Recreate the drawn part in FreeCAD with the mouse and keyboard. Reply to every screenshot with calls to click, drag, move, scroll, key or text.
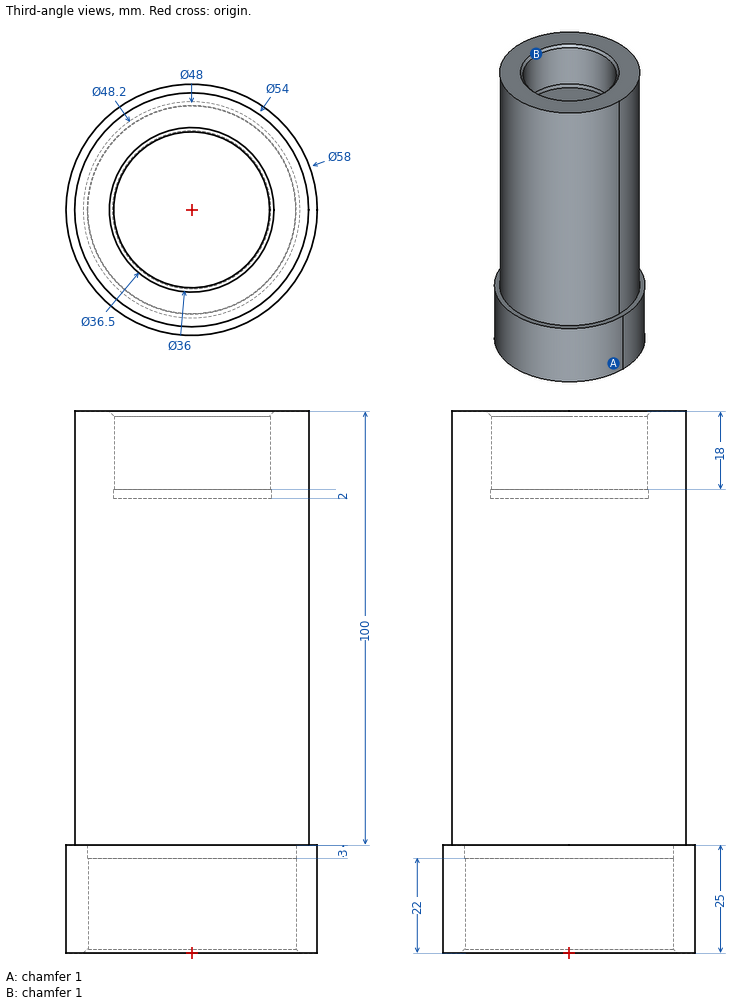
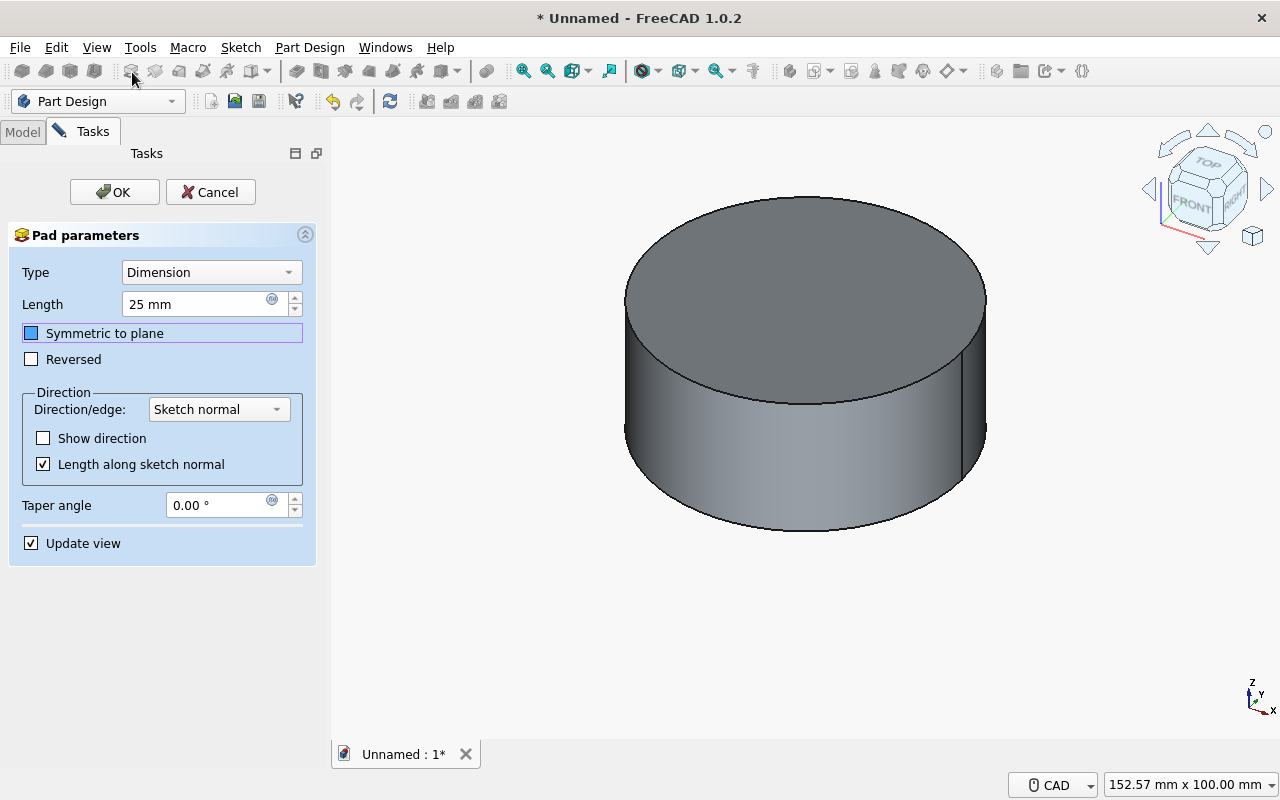
click(115, 192)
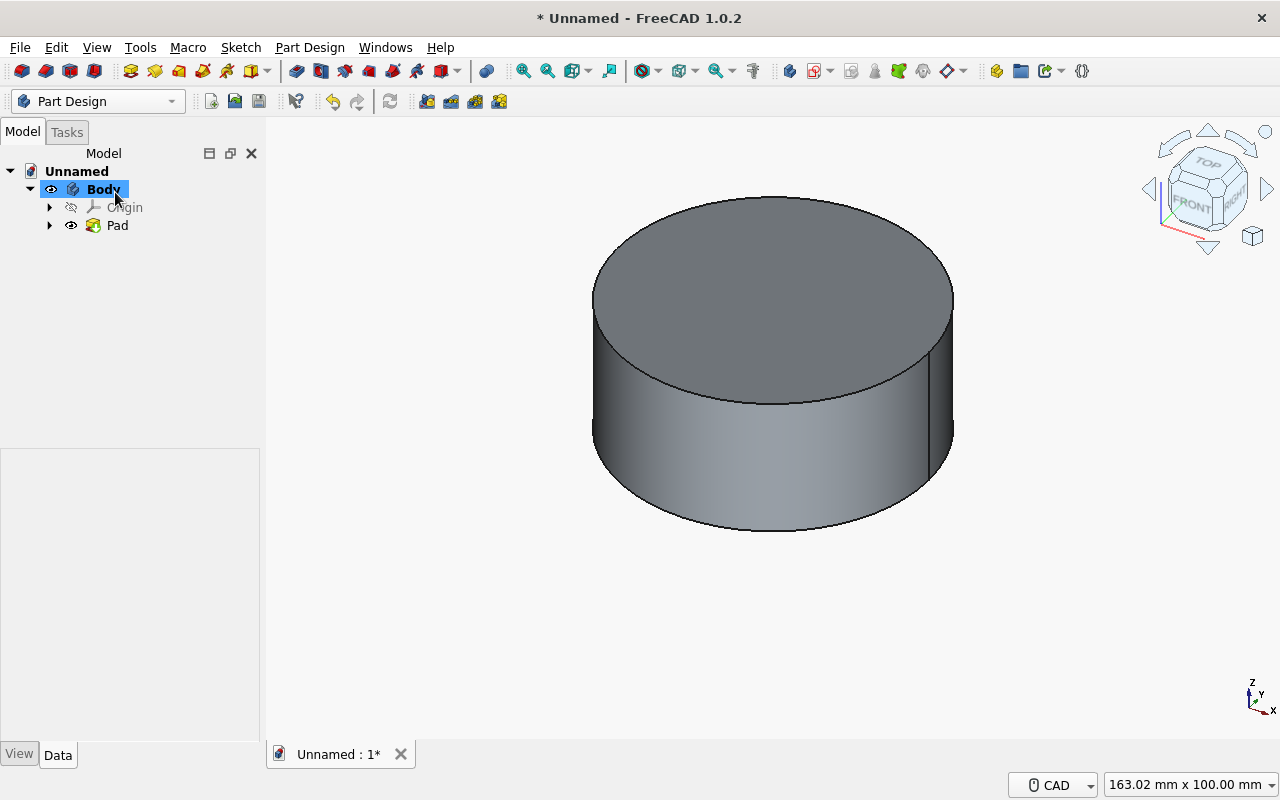
click(773, 300)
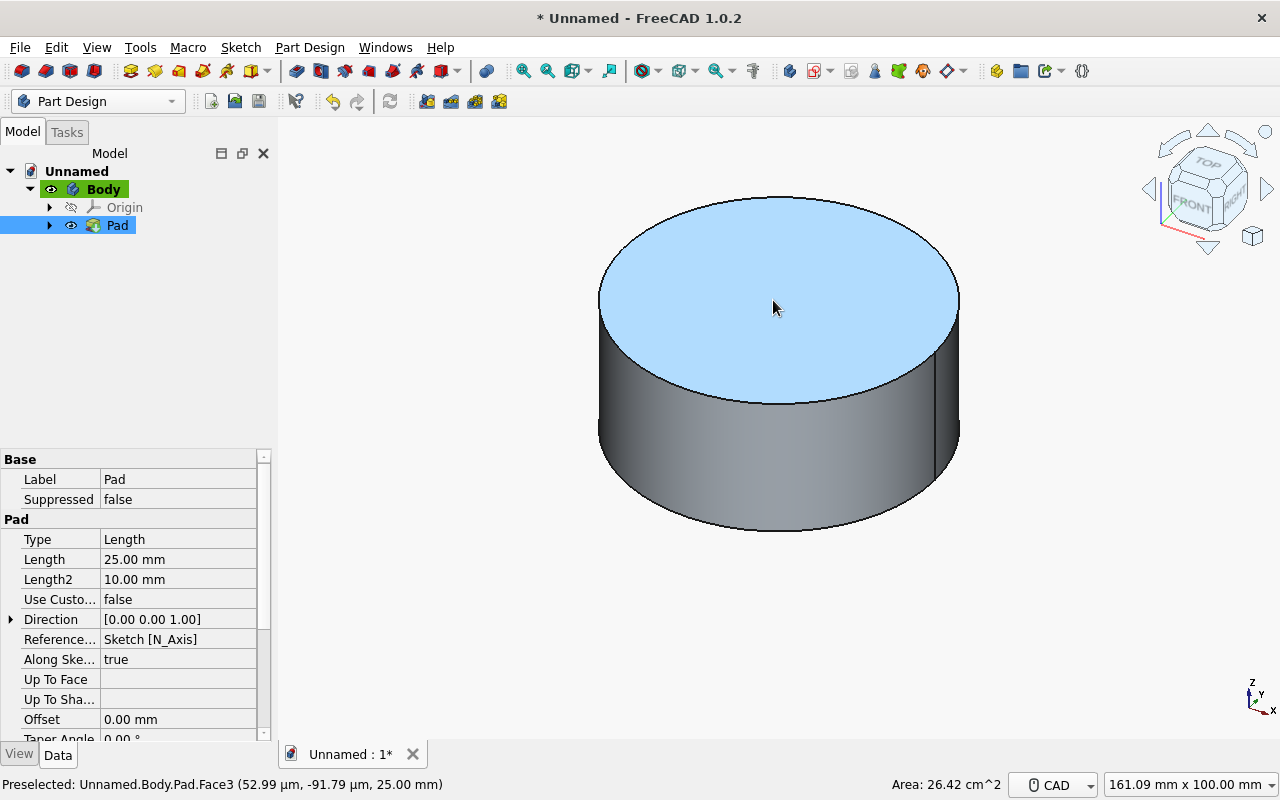
click(814, 72)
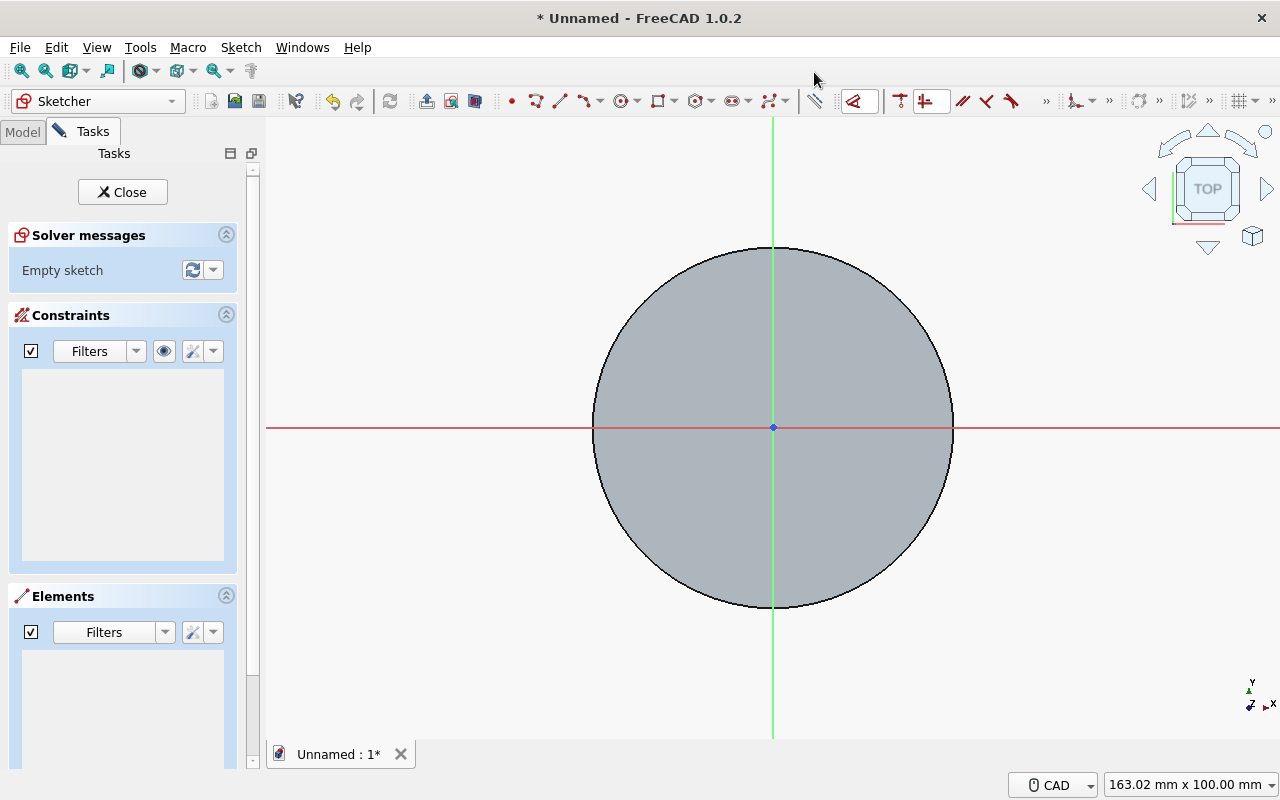
click(622, 102)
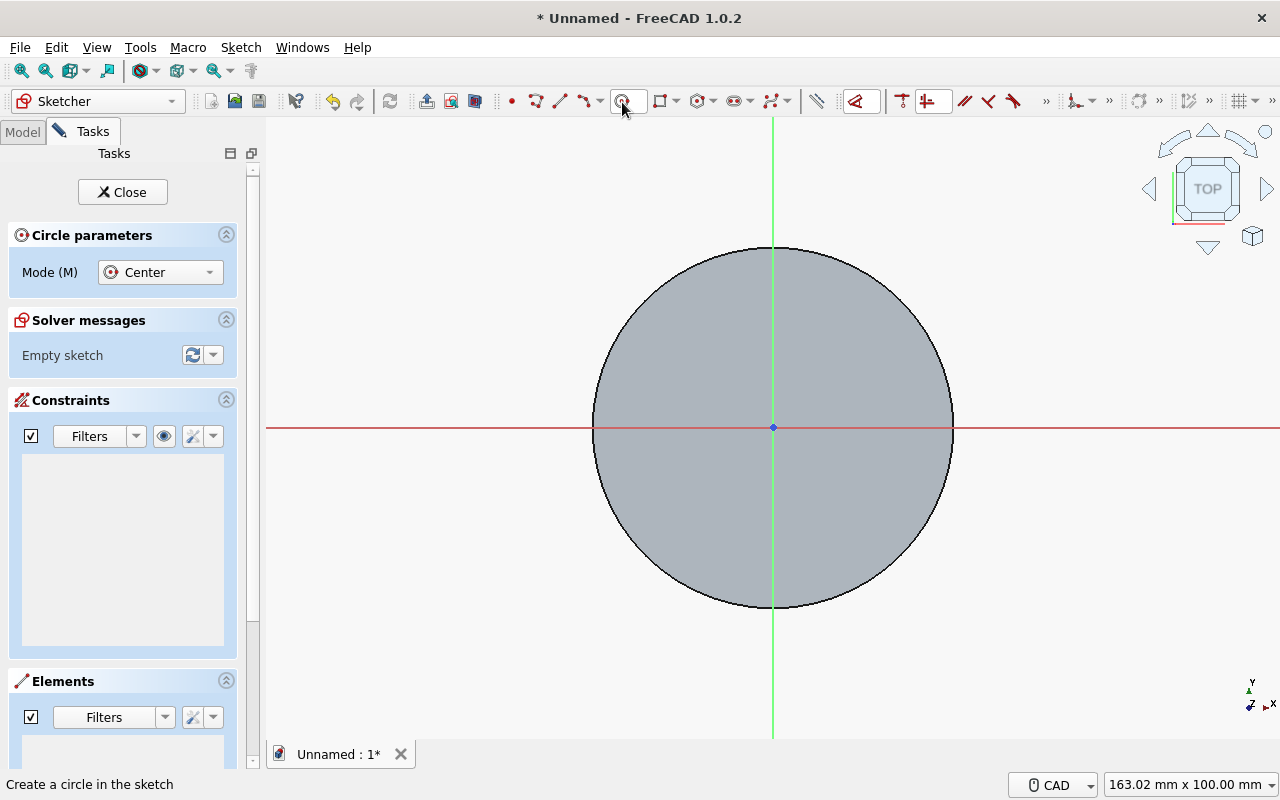
click(773, 428)
move(892, 309)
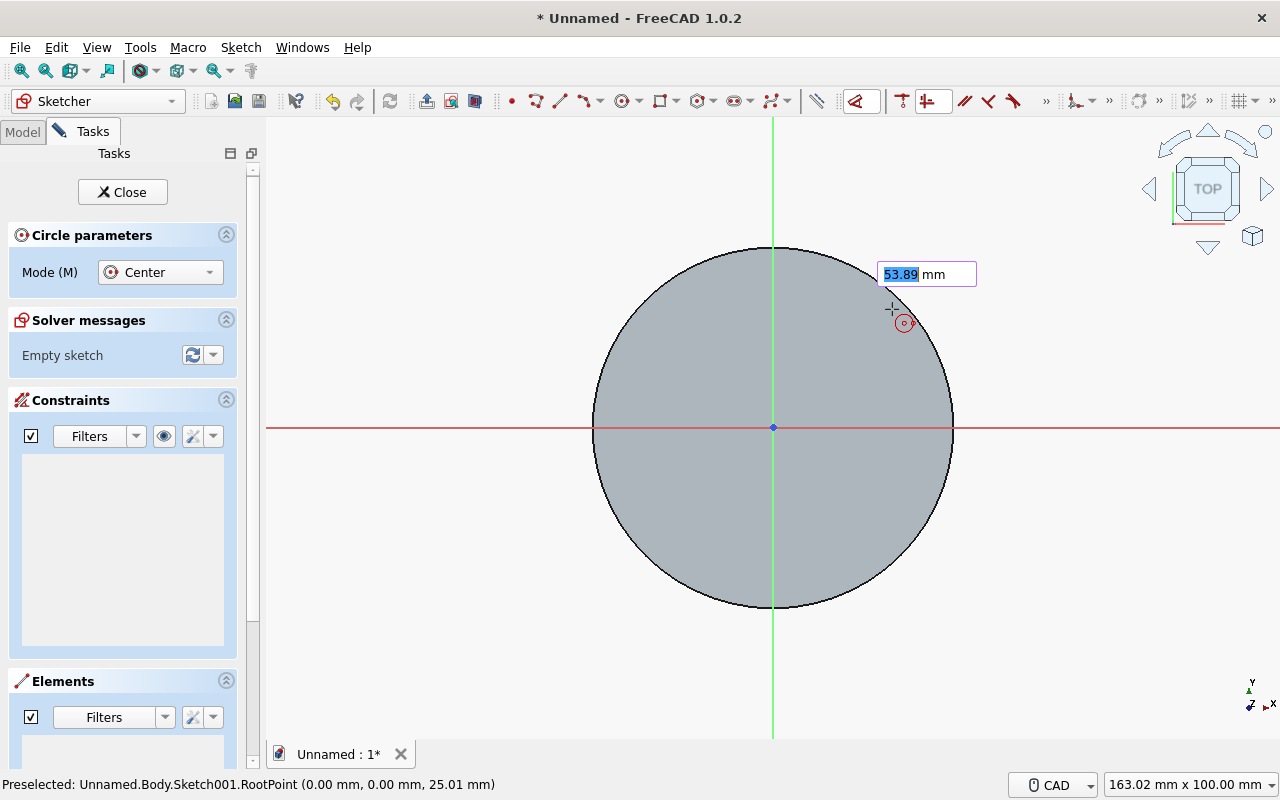
text(54)
key(Return)
key(Escape)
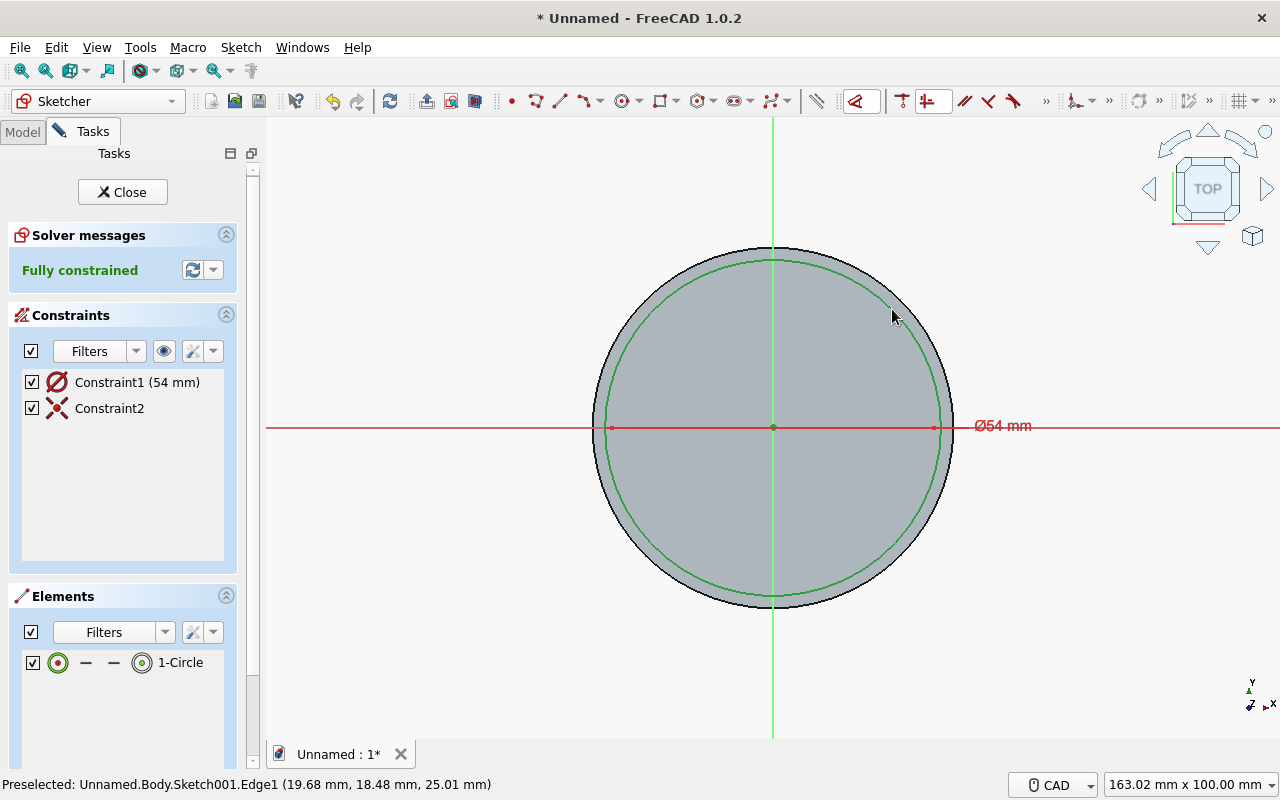
click(123, 192)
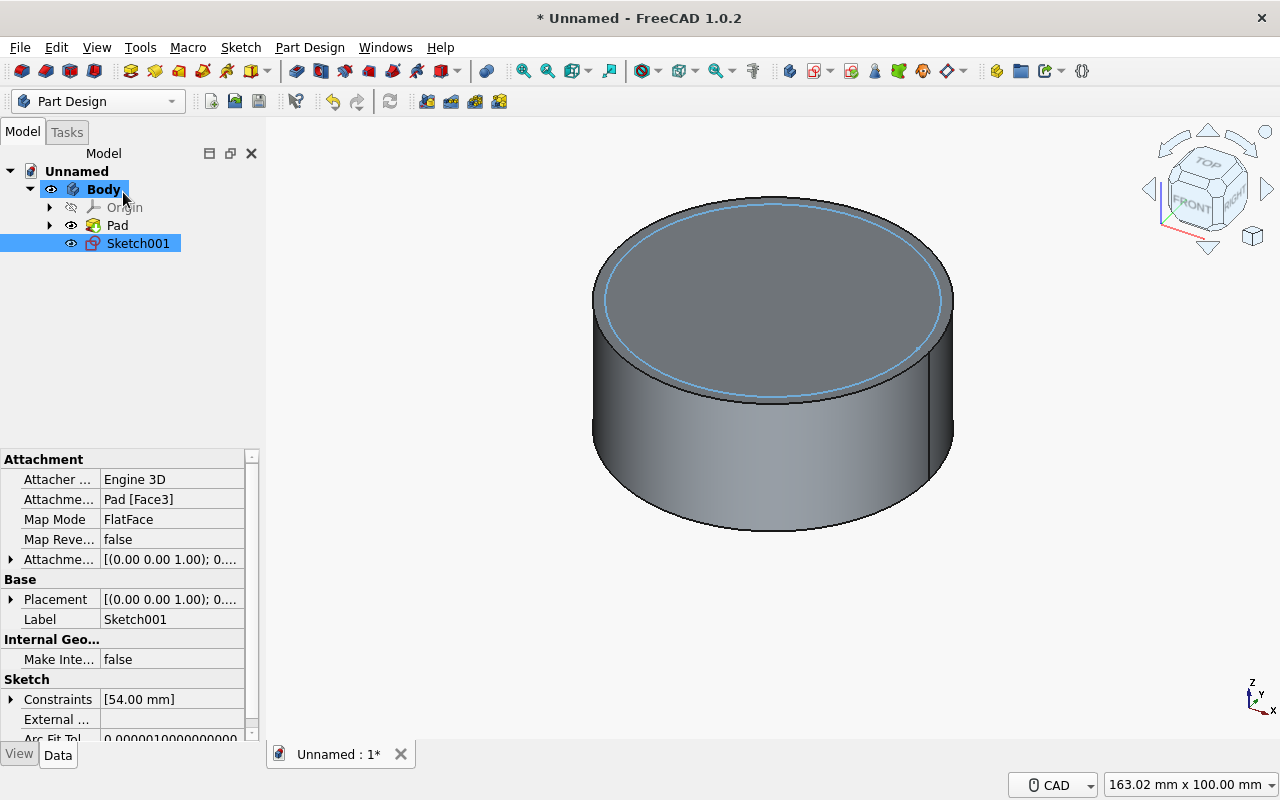
click(132, 72)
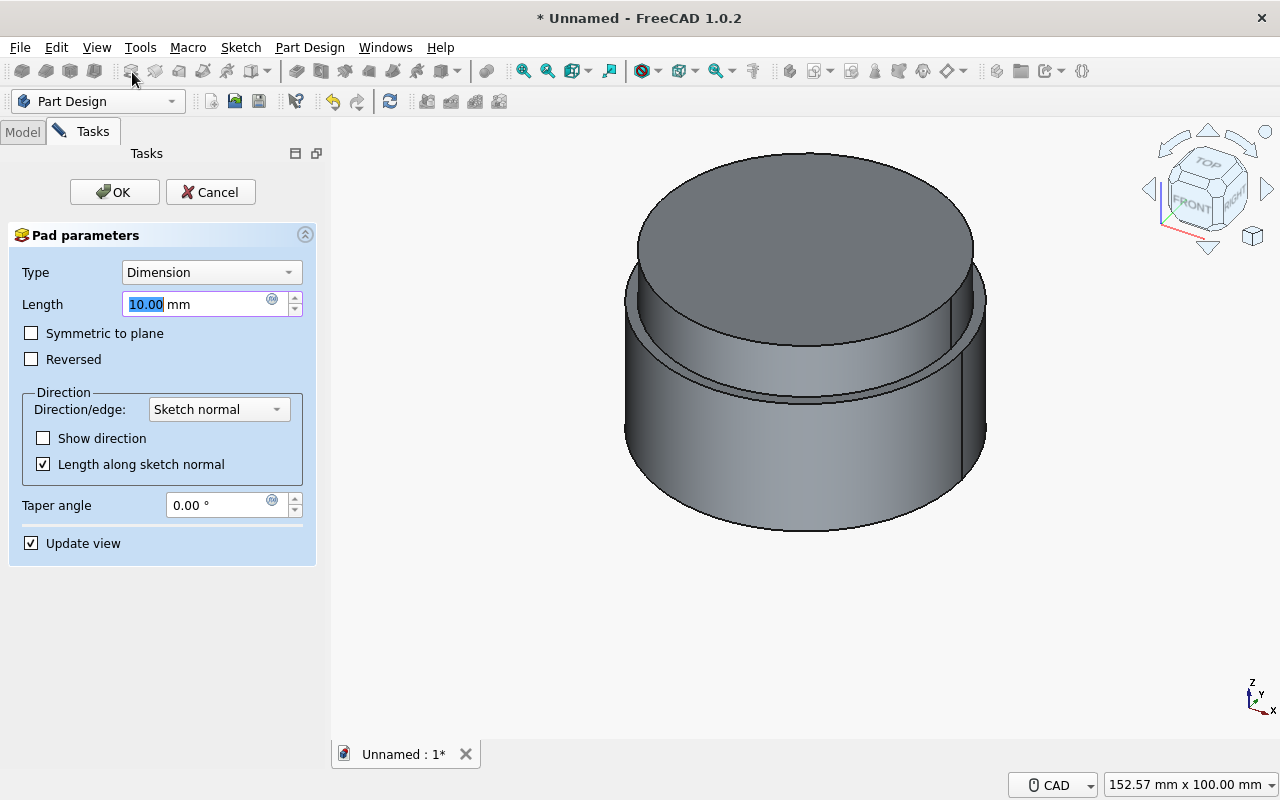
text(100)
key(Tab)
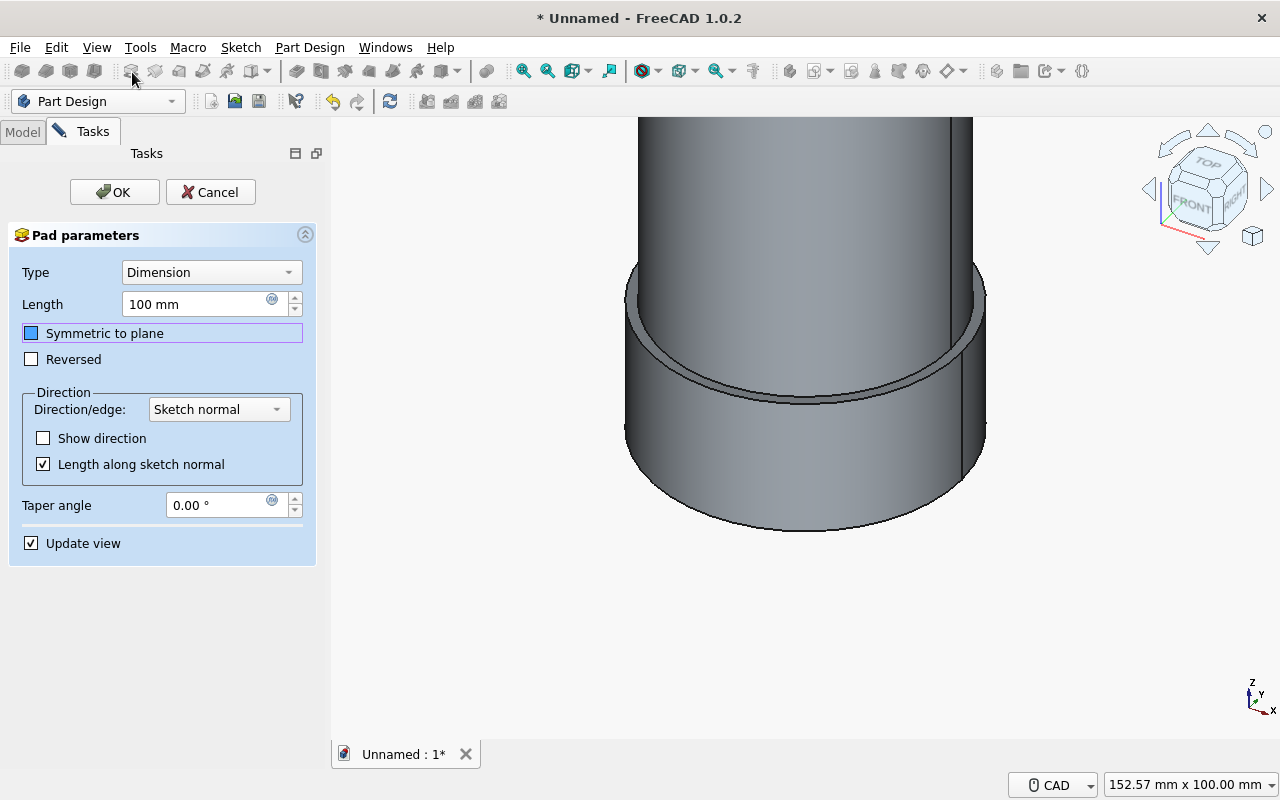
click(115, 192)